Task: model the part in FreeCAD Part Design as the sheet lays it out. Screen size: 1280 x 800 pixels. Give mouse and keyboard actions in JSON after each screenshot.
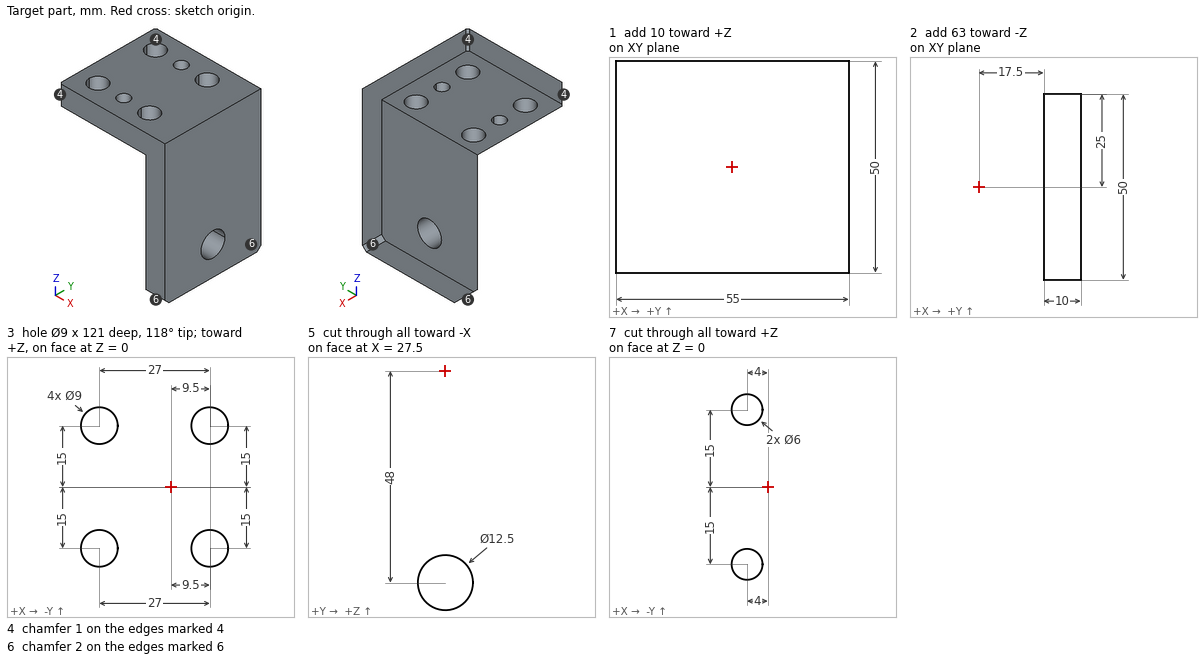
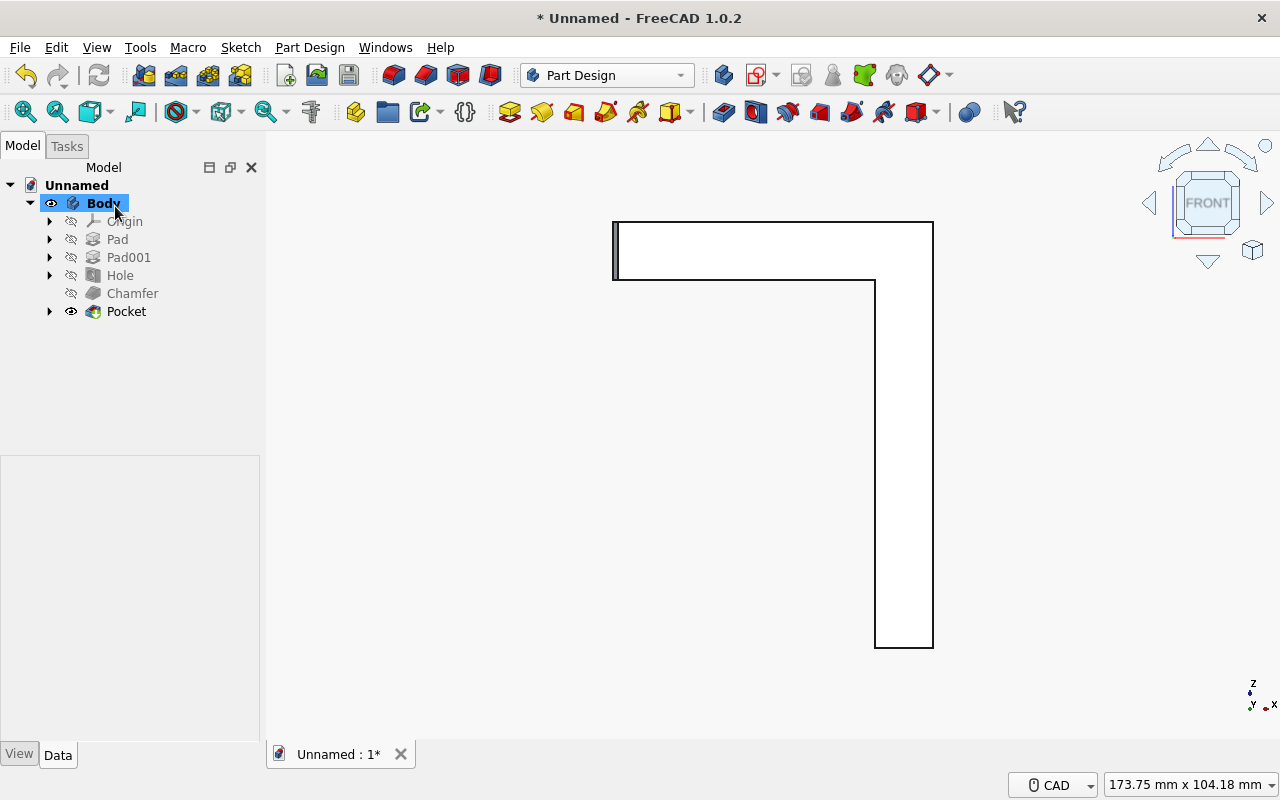
{"action": "left_click", "coordinate": [904, 647]}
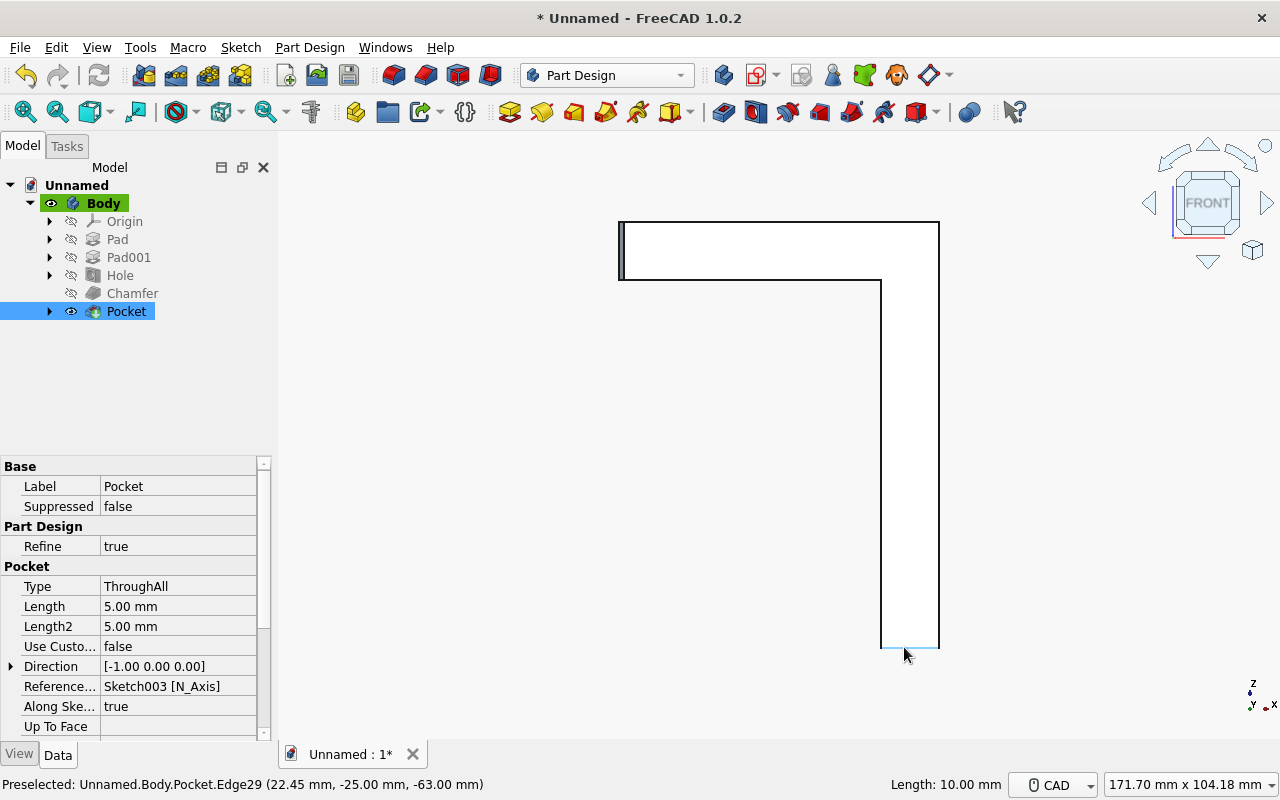
{"action": "key", "text": "3"}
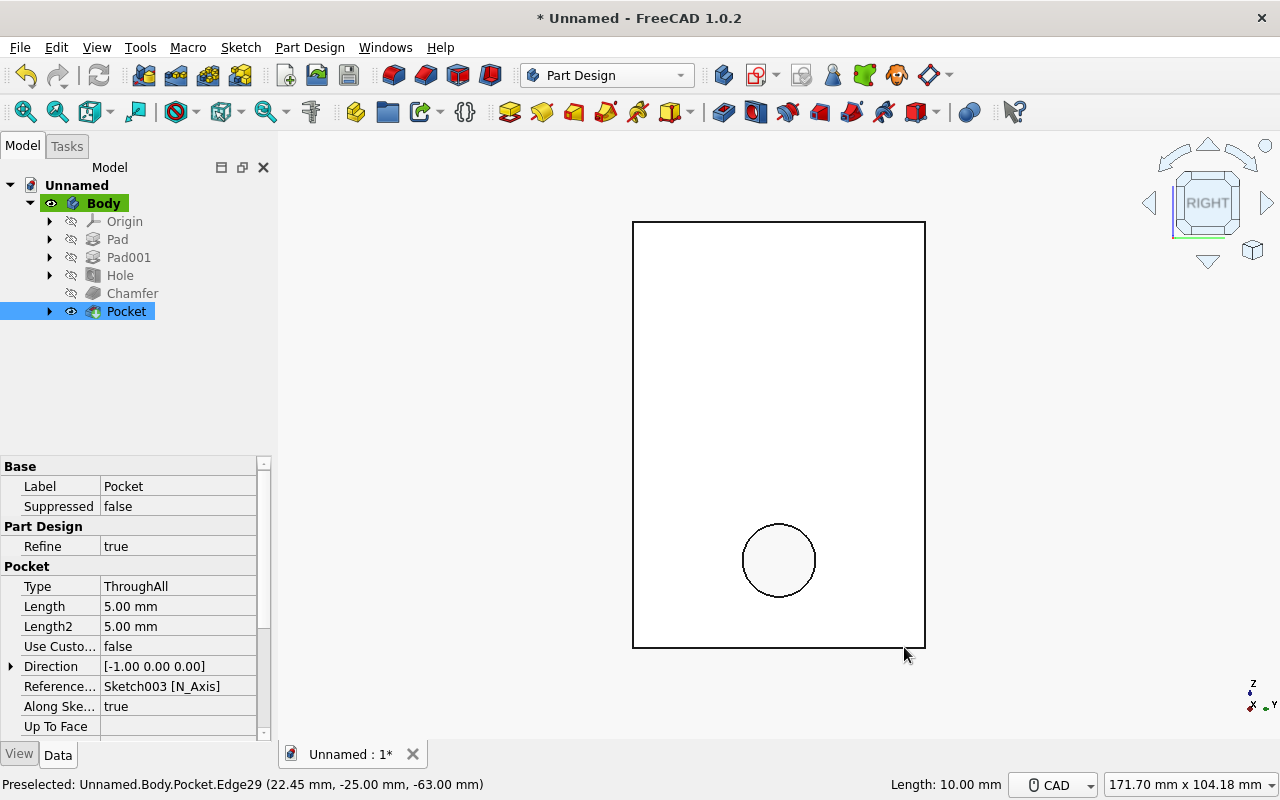
{"action": "key", "text": "5"}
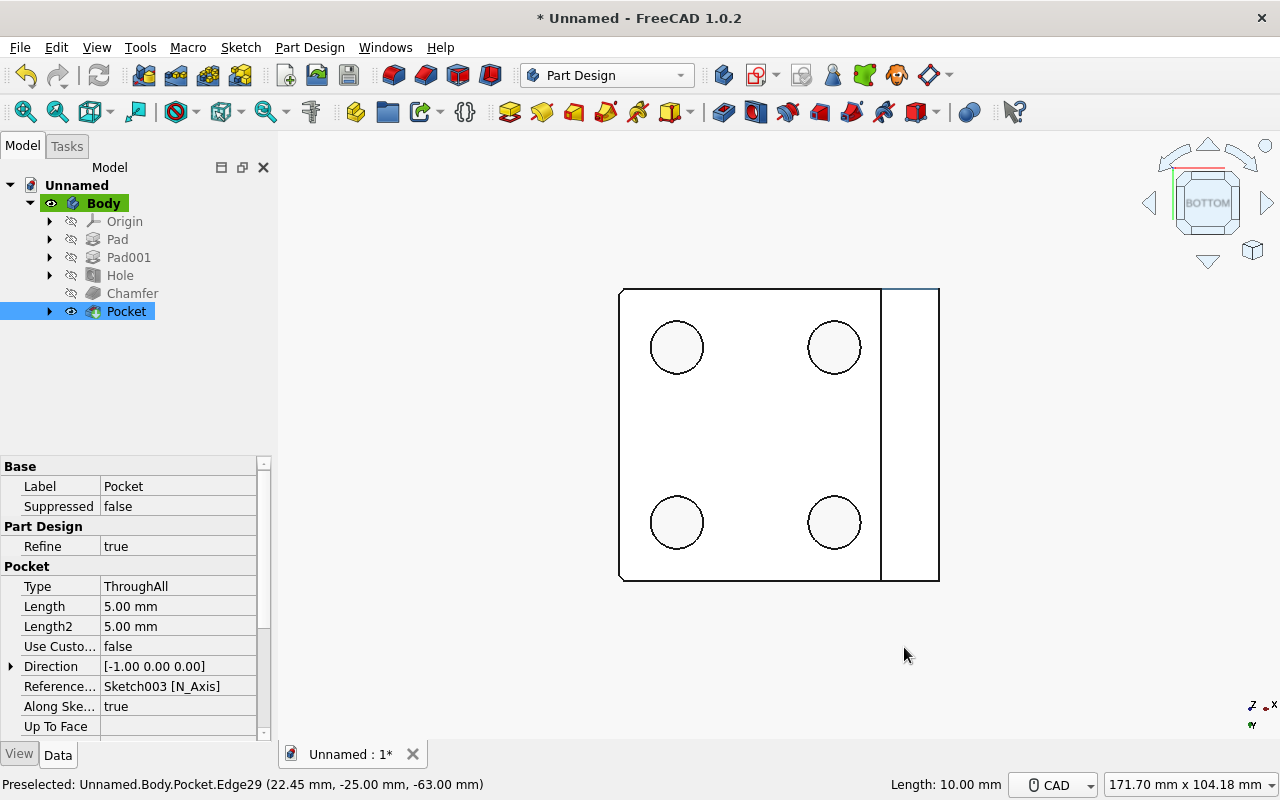
{"action": "left_click", "coordinate": [910, 580], "text": "ctrl"}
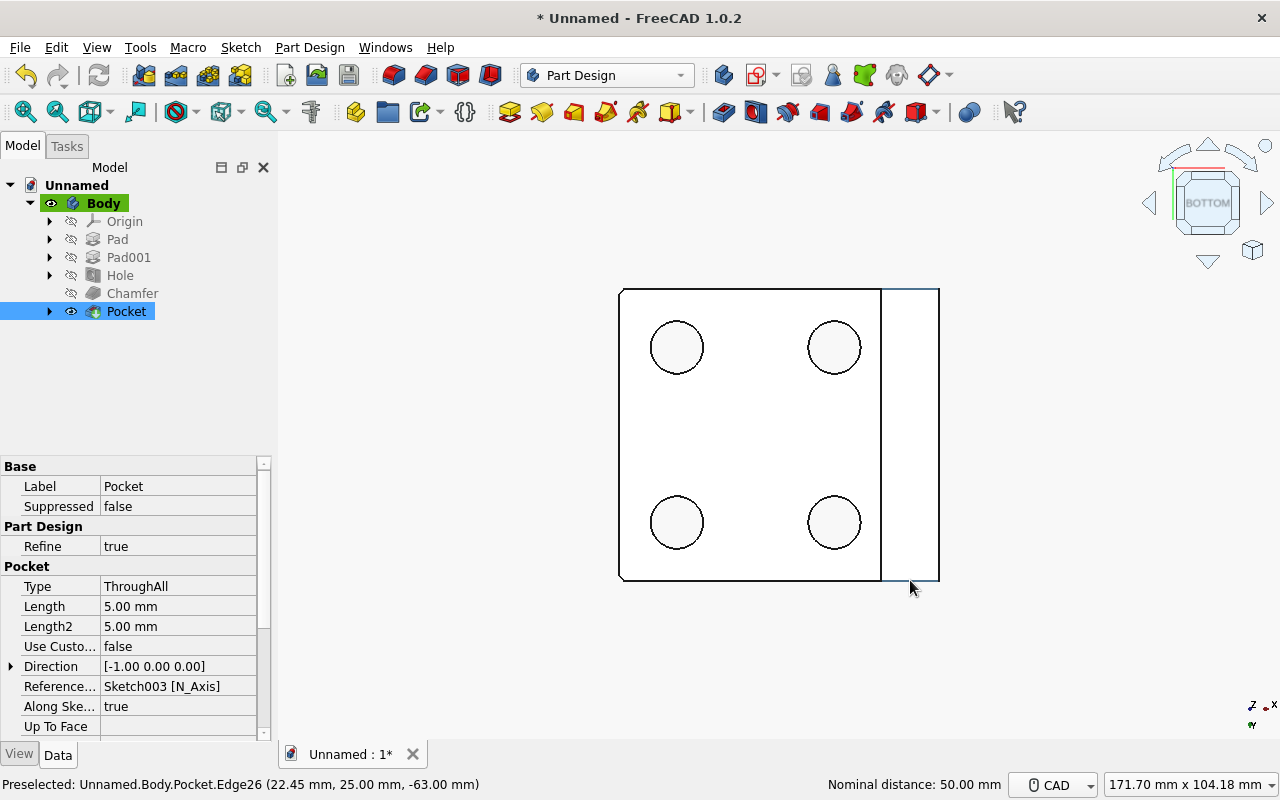
{"action": "left_click", "coordinate": [426, 76]}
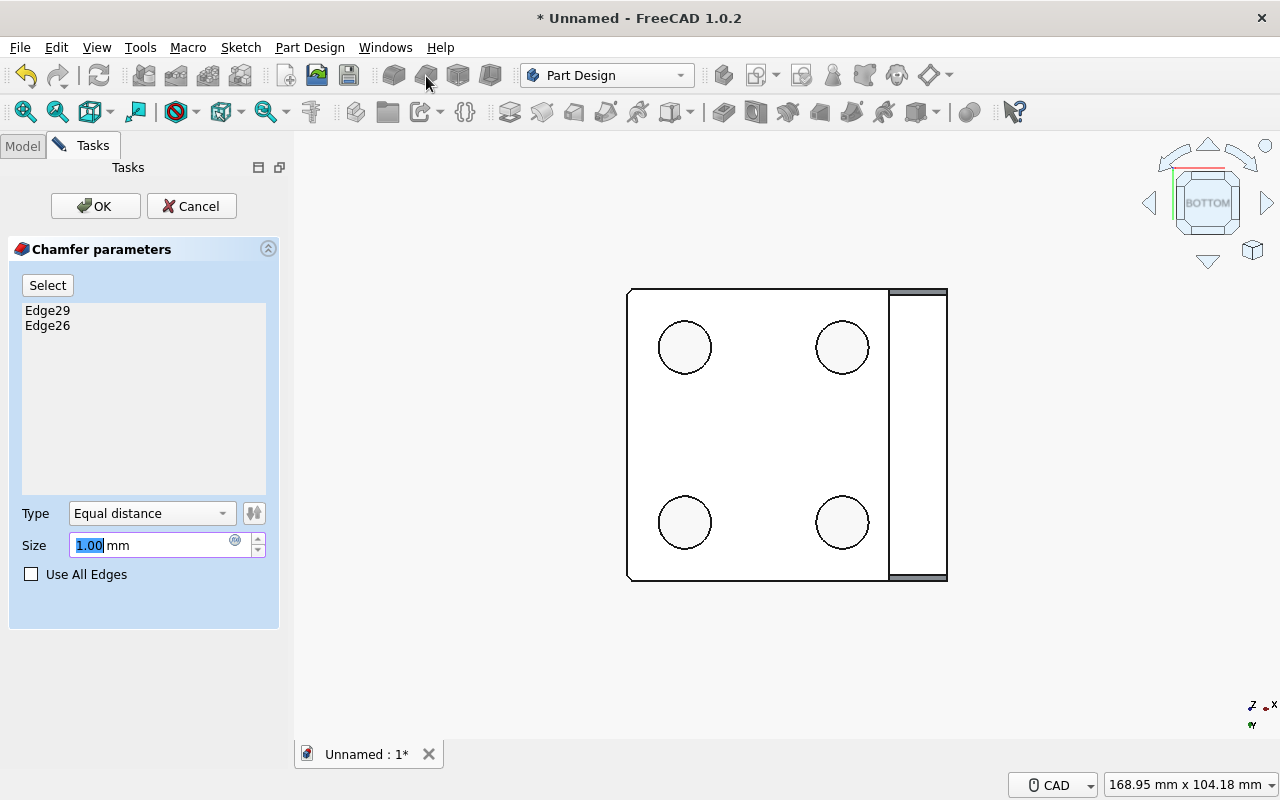
{"action": "type", "text": "2"}
{"action": "key", "text": "Tab"}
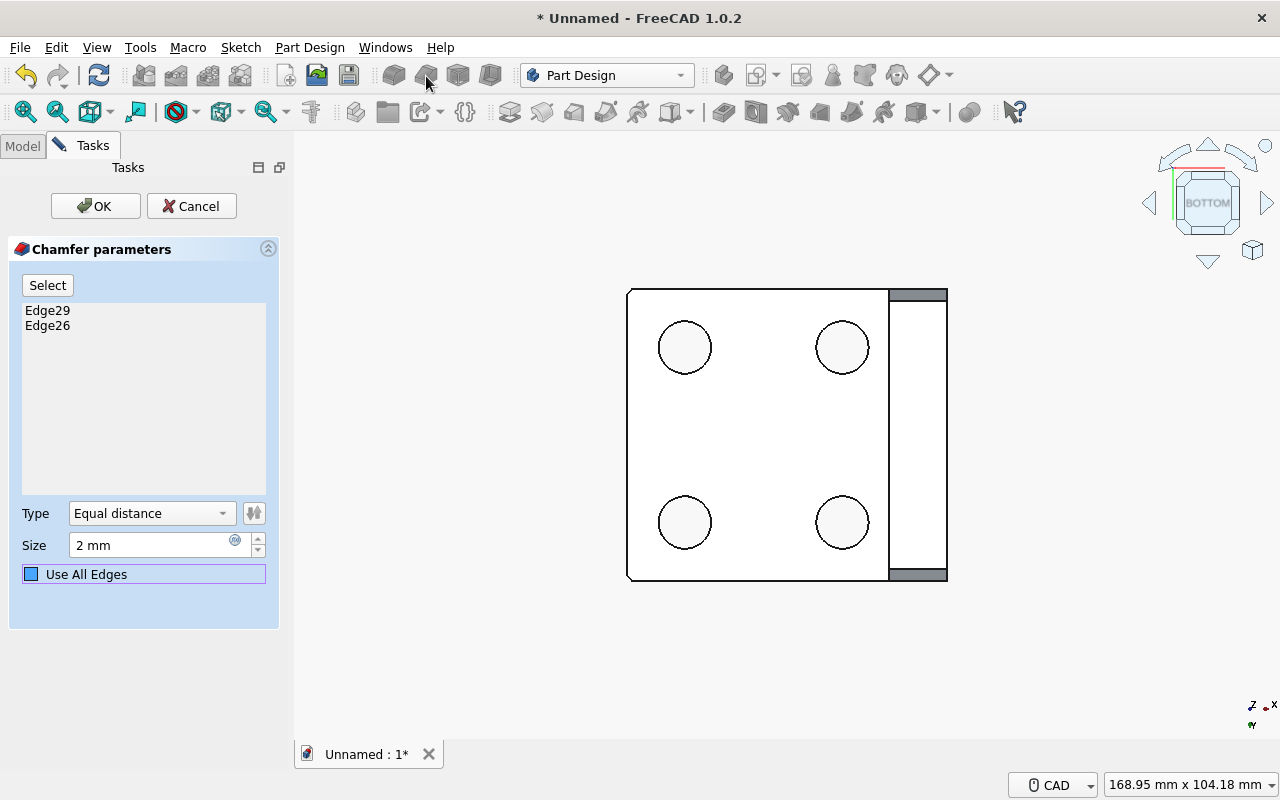
{"action": "left_click", "coordinate": [96, 206]}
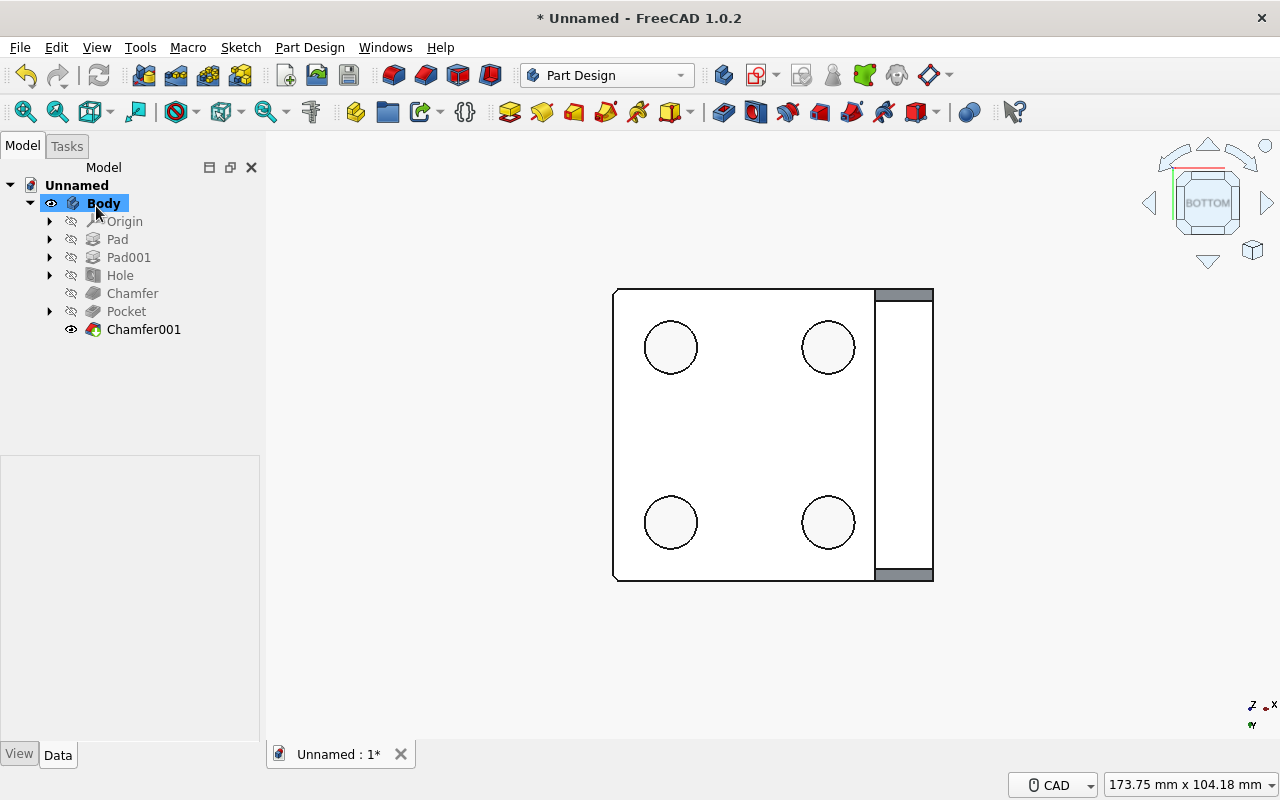
{"action": "left_click", "coordinate": [744, 434]}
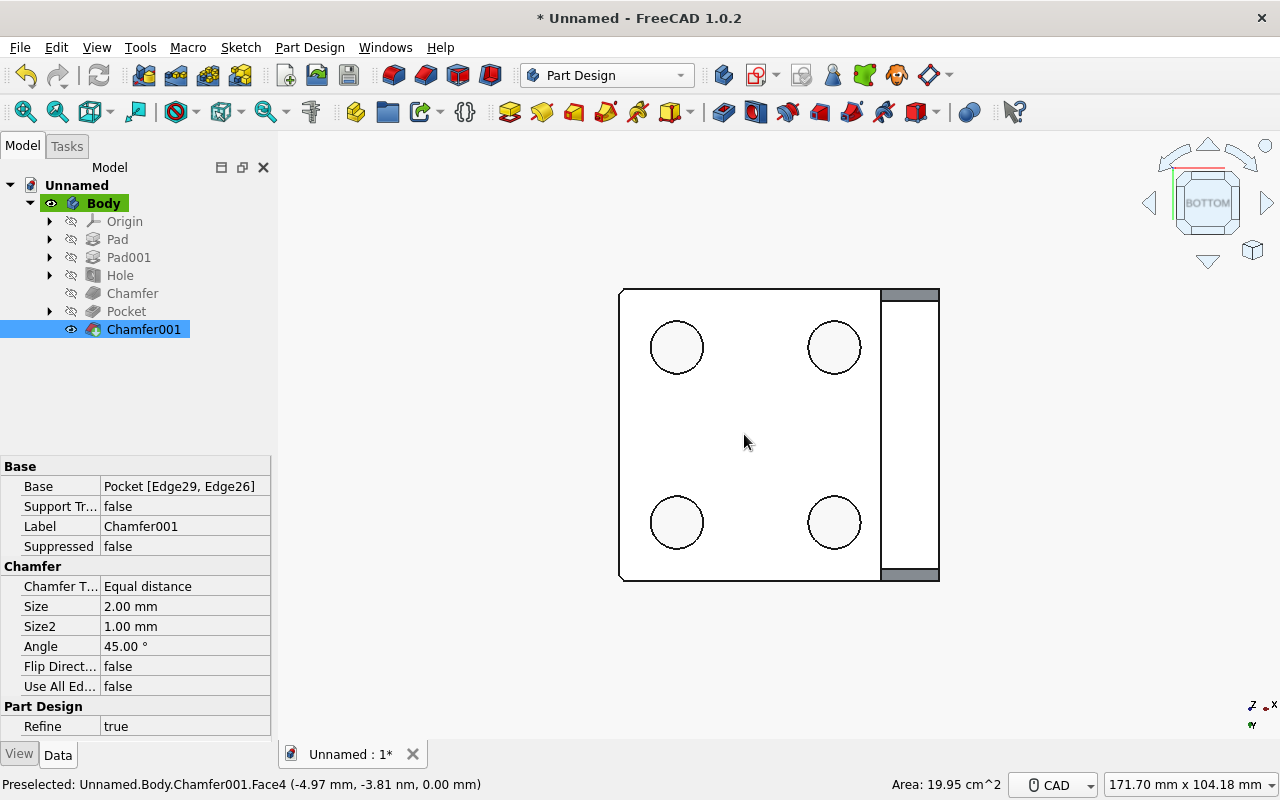
{"action": "left_click", "coordinate": [756, 76]}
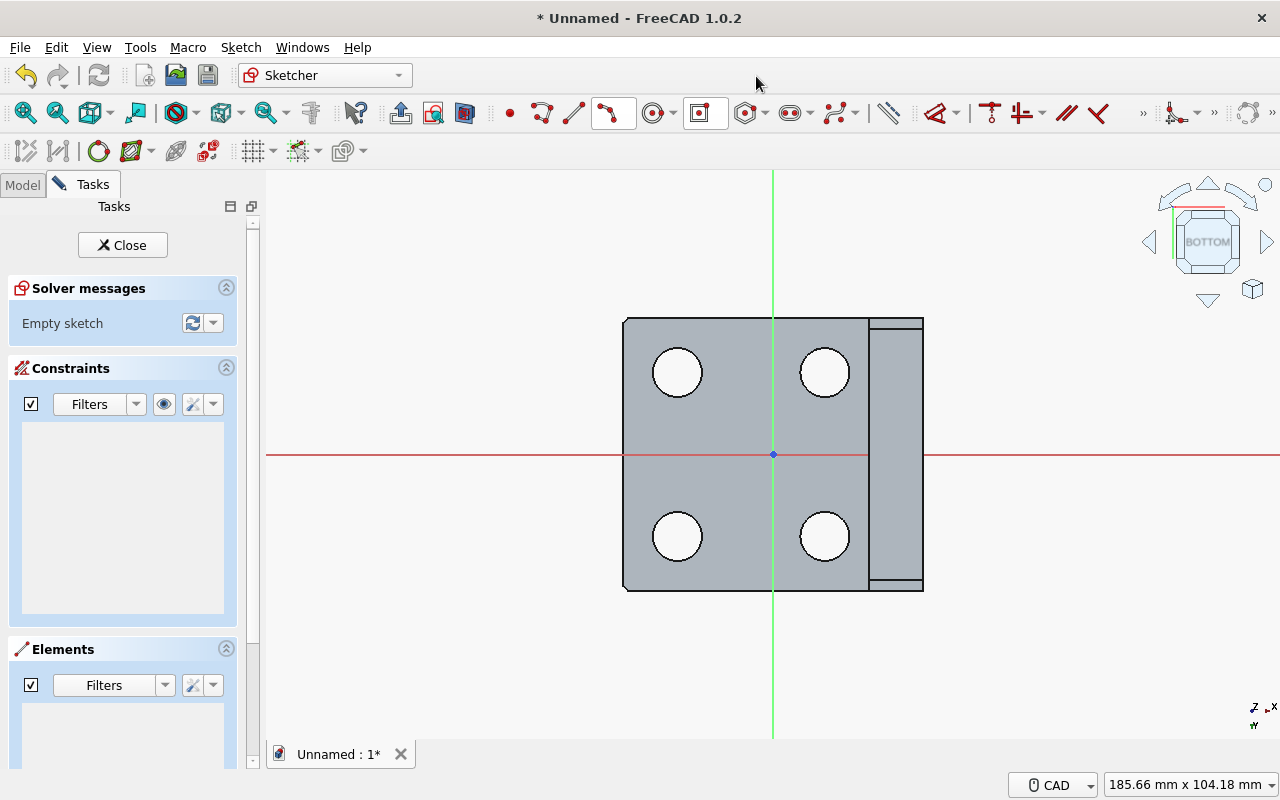
{"action": "left_click", "coordinate": [466, 114]}